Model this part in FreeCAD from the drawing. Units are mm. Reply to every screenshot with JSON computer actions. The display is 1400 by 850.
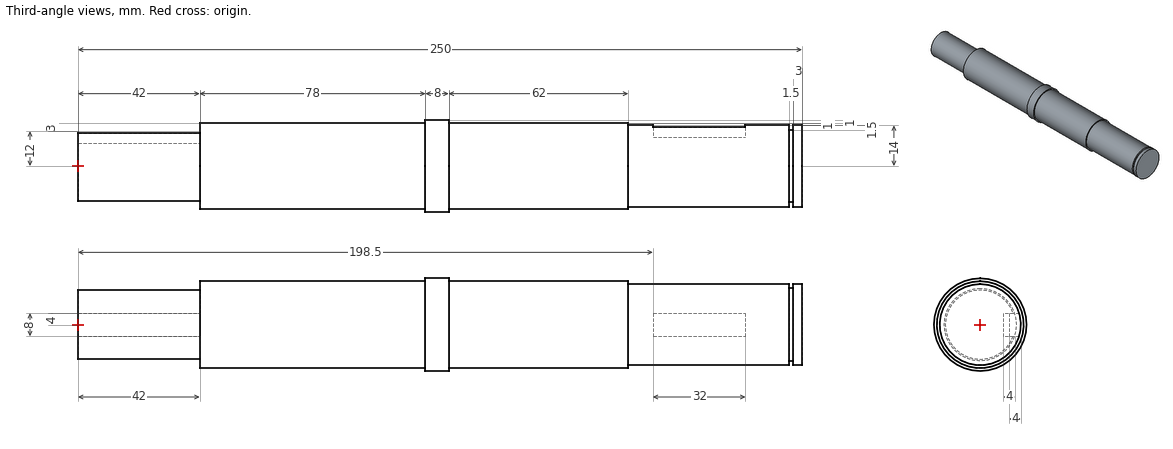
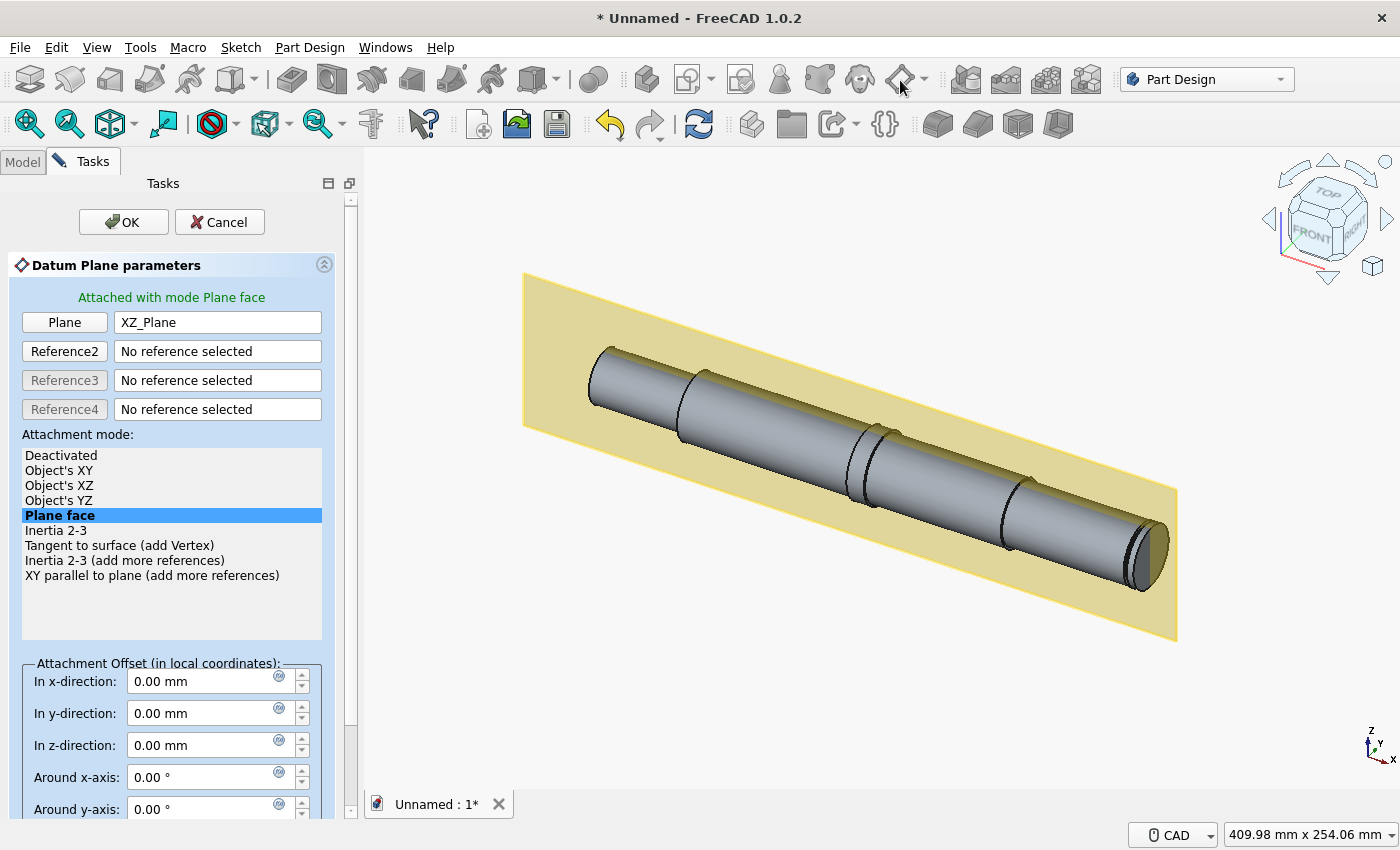
{"action": "triple_click", "coordinate": [210, 745]}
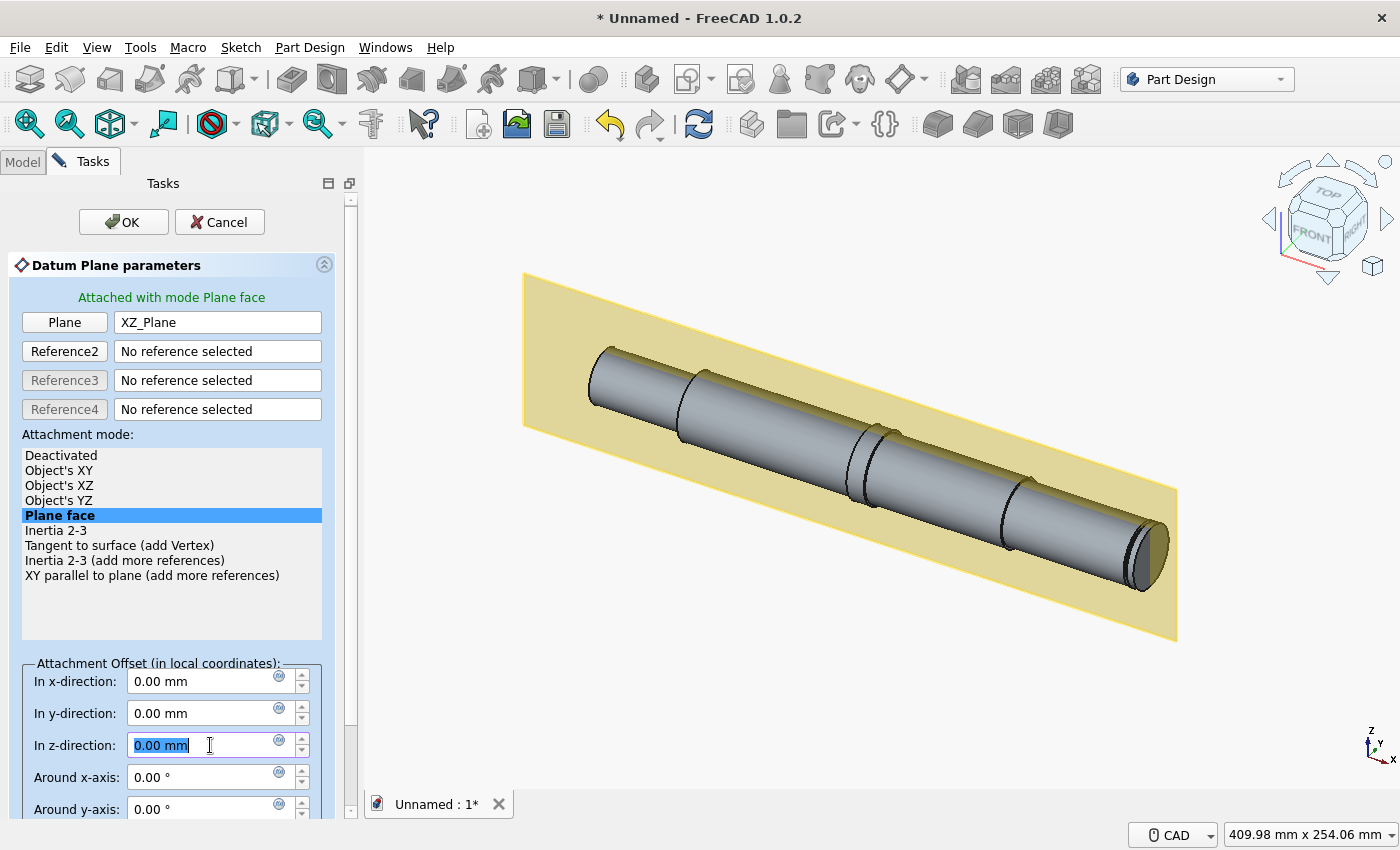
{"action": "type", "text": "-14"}
{"action": "key", "text": "Tab"}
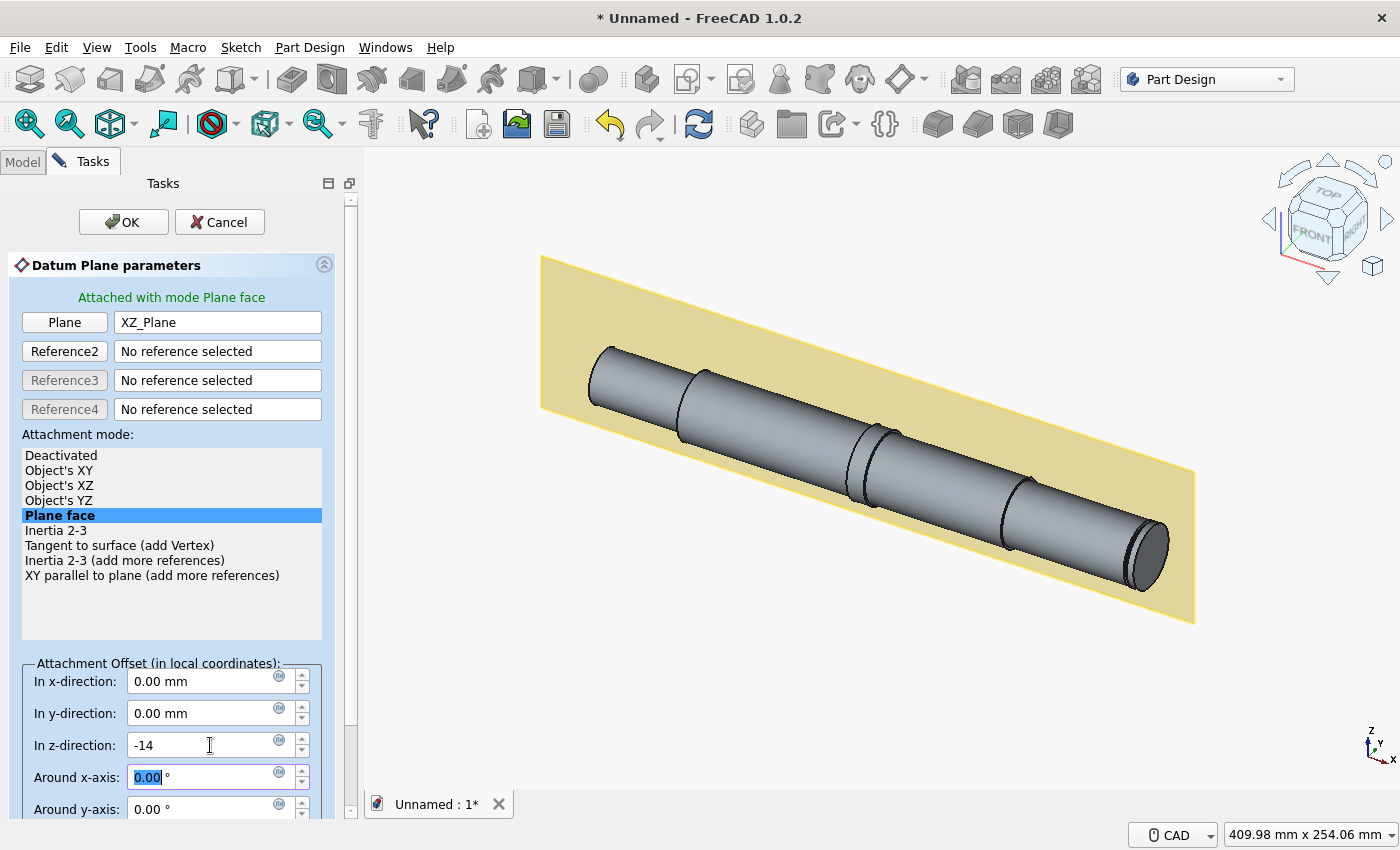
{"action": "left_click", "coordinate": [124, 222]}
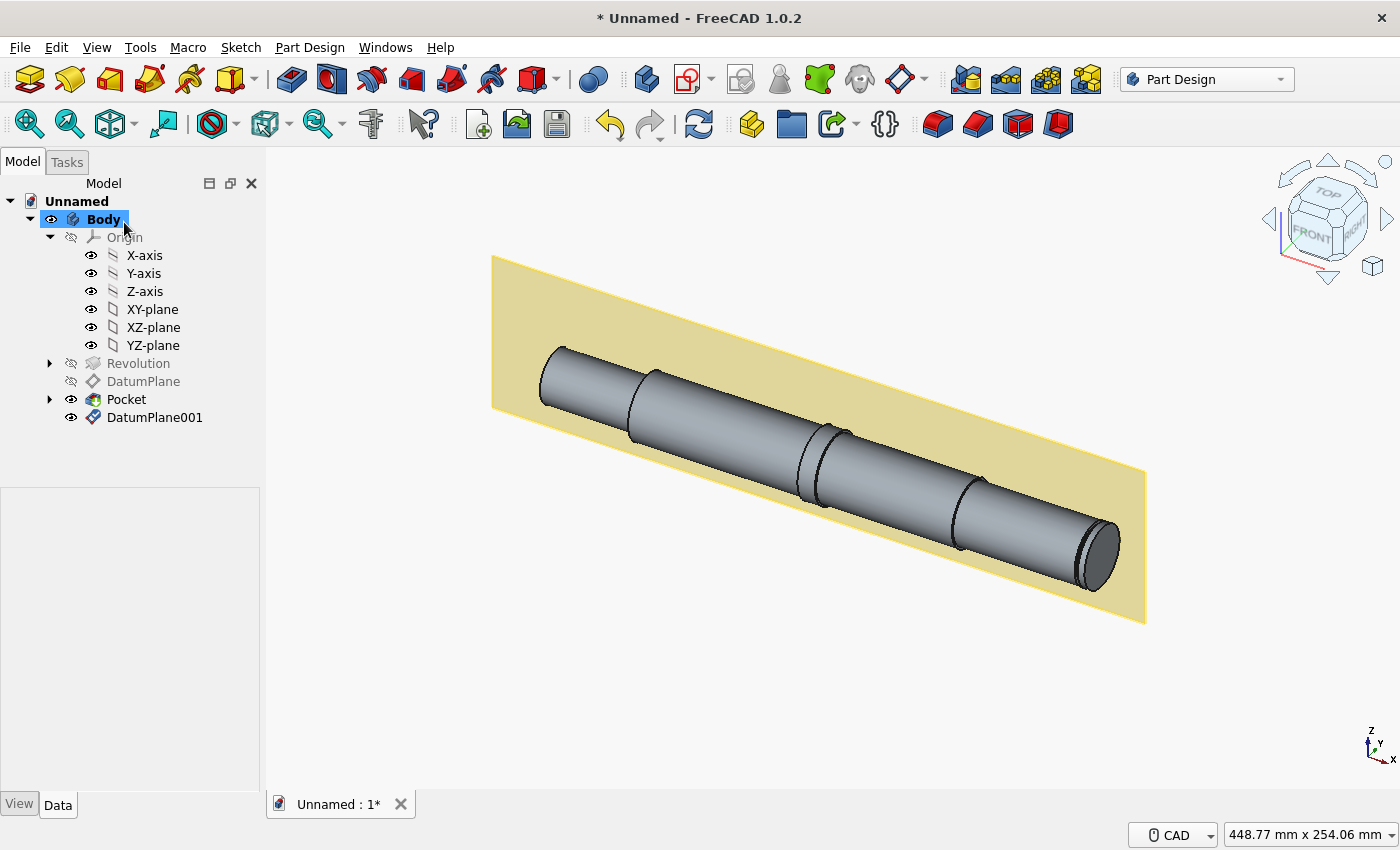
{"action": "left_click", "coordinate": [116, 417]}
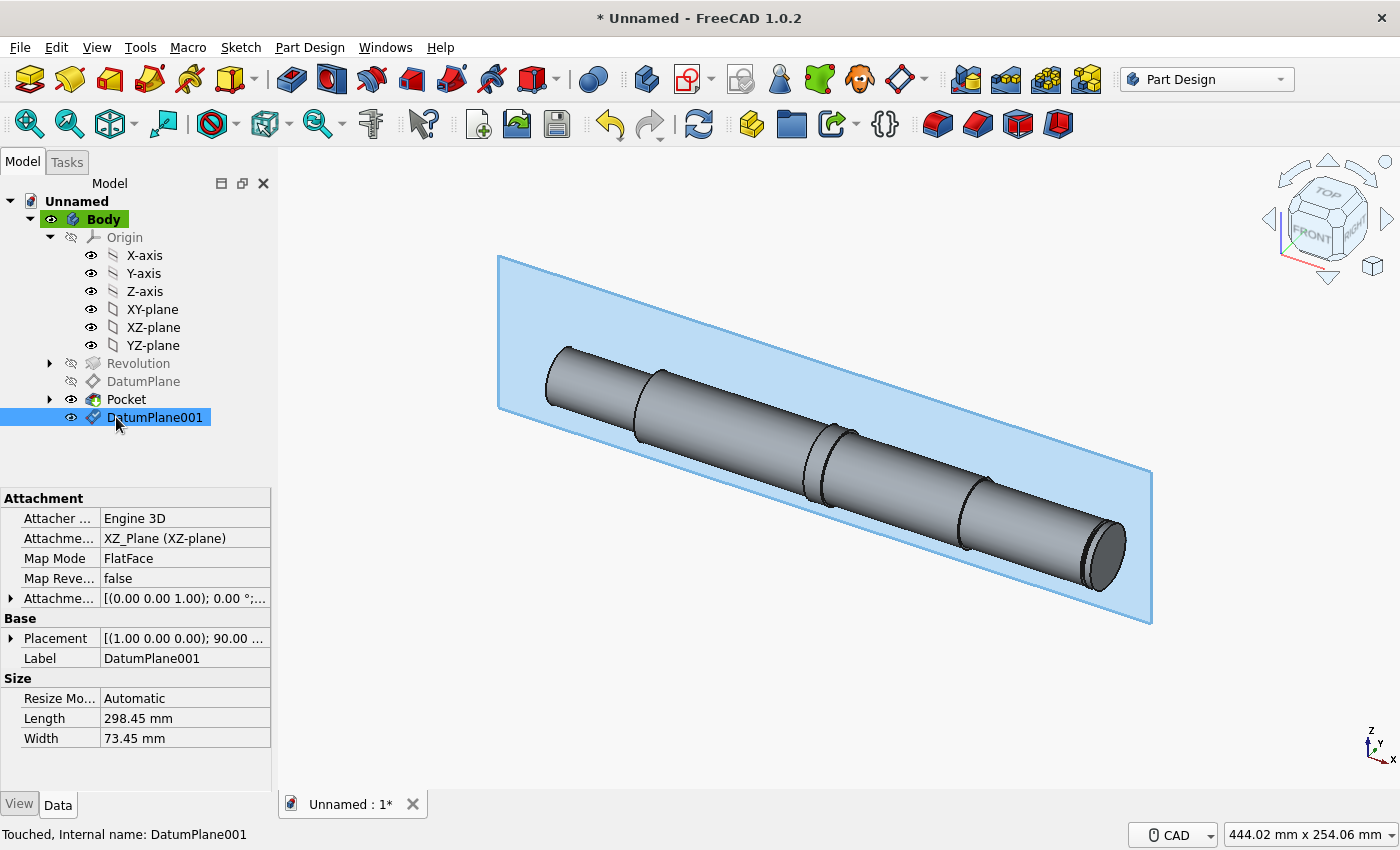
{"action": "left_click", "coordinate": [688, 80]}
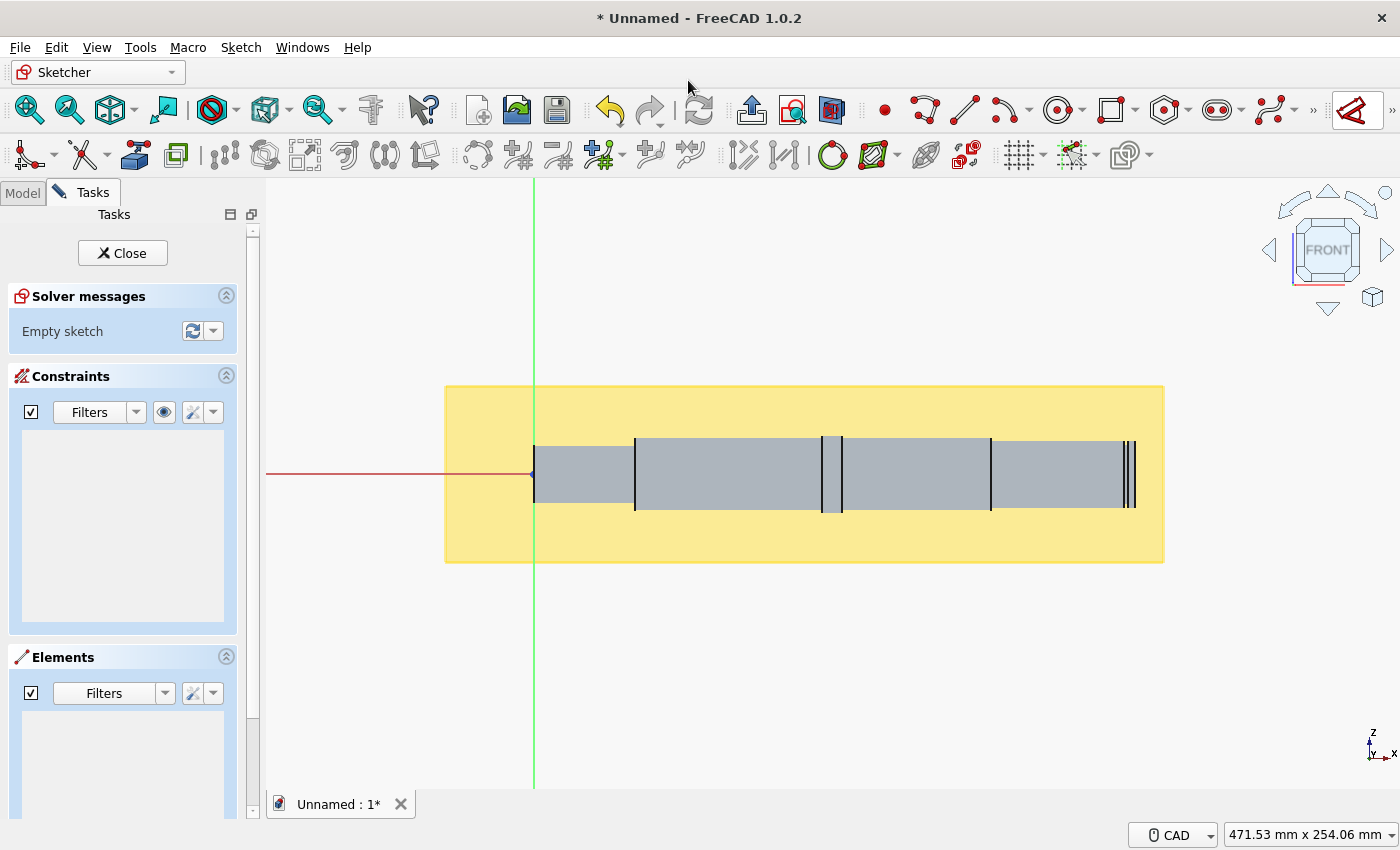
{"action": "left_click", "coordinate": [832, 110]}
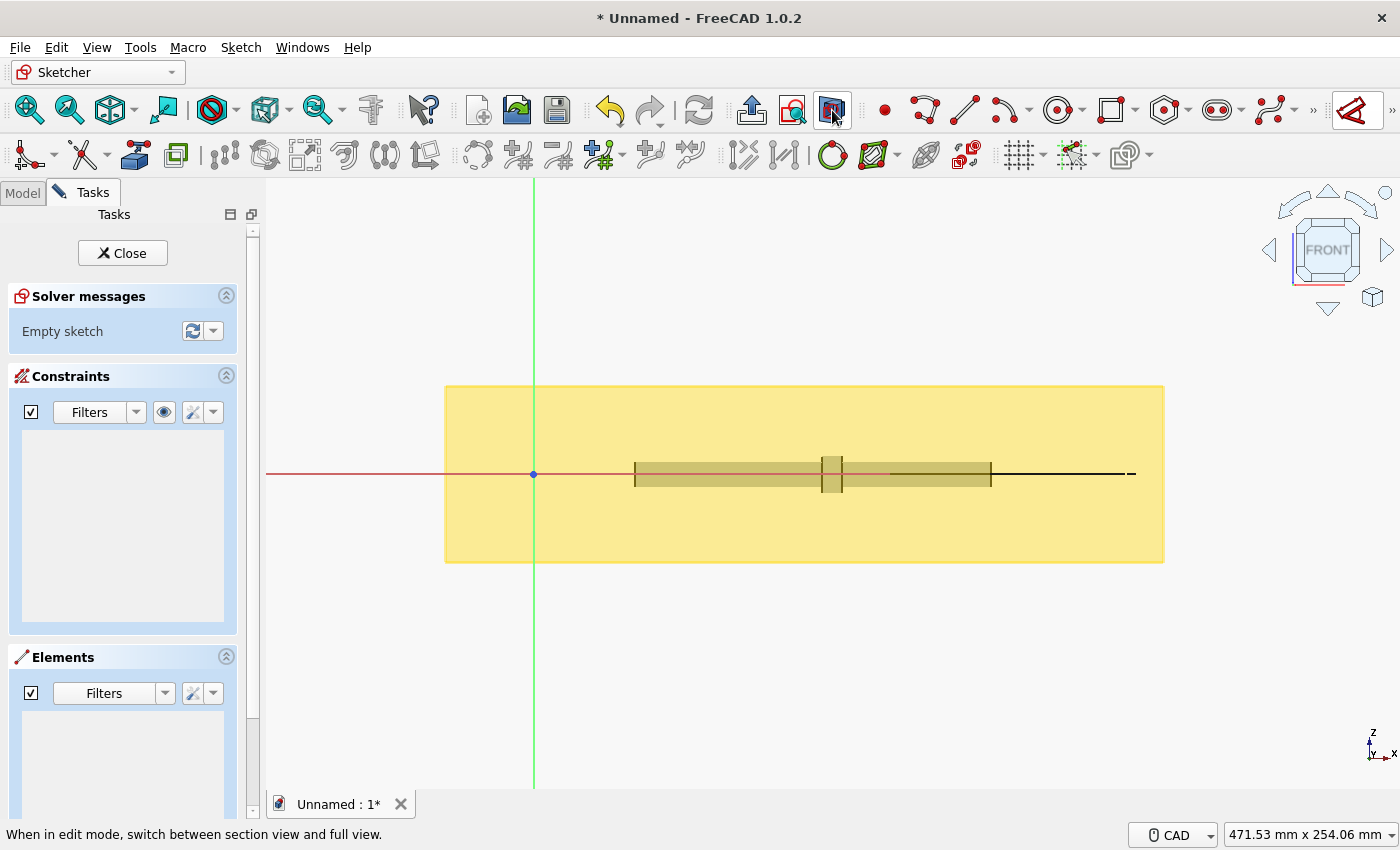
{"action": "scroll", "coordinate": [1085, 473], "scroll_direction": "up", "scroll_amount": 11}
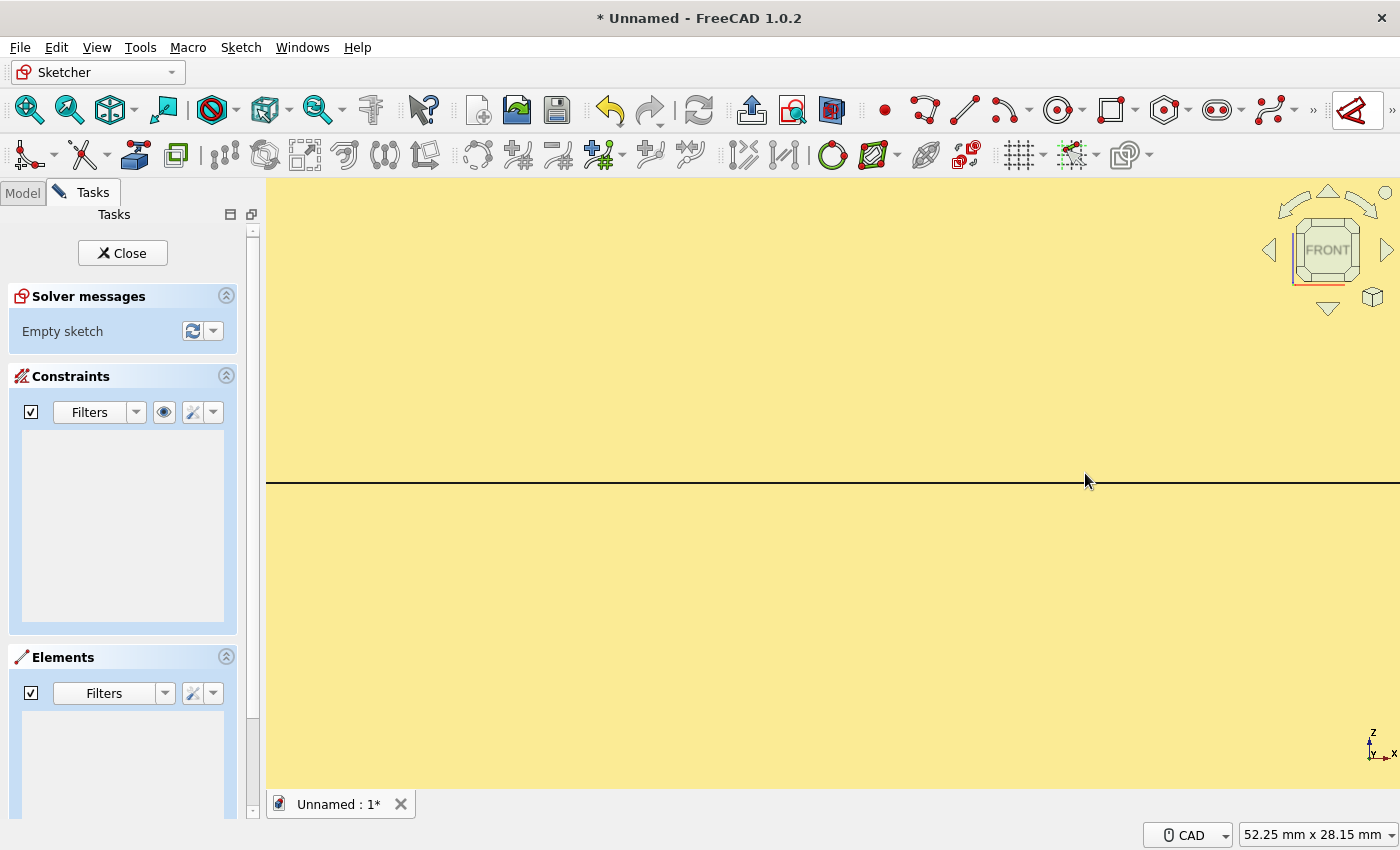
{"action": "left_click", "coordinate": [1112, 110]}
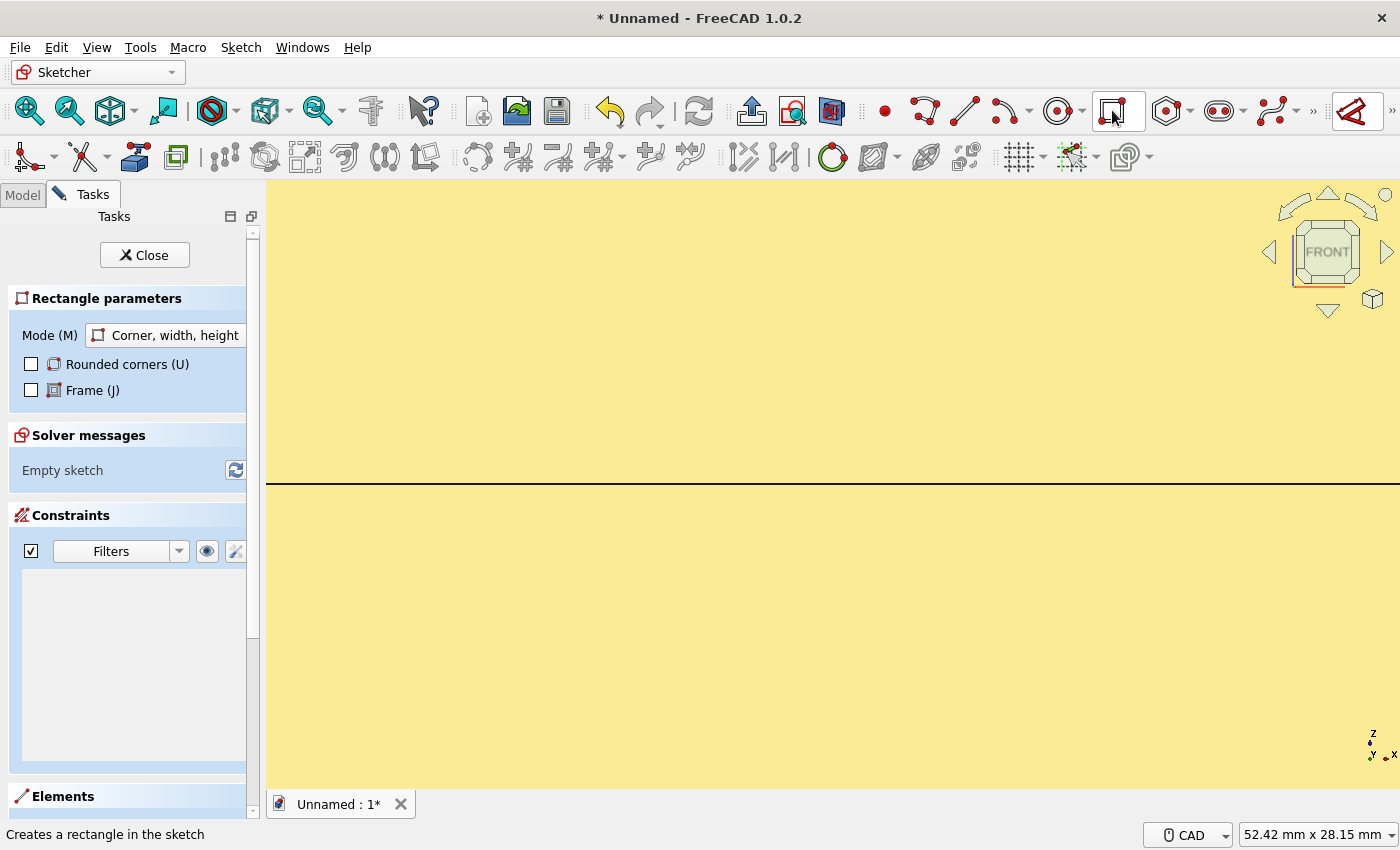
{"action": "left_click", "coordinate": [415, 397]}
{"action": "mouse_move", "coordinate": [1107, 570]}